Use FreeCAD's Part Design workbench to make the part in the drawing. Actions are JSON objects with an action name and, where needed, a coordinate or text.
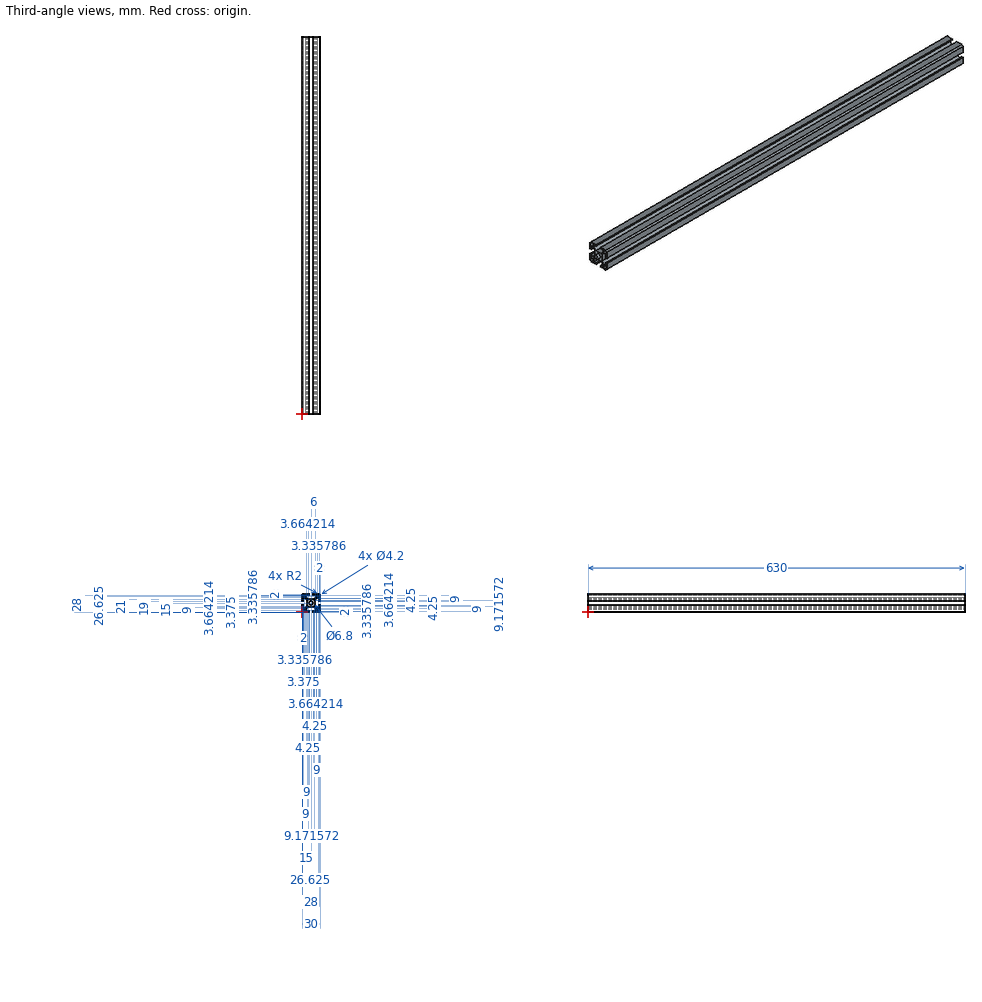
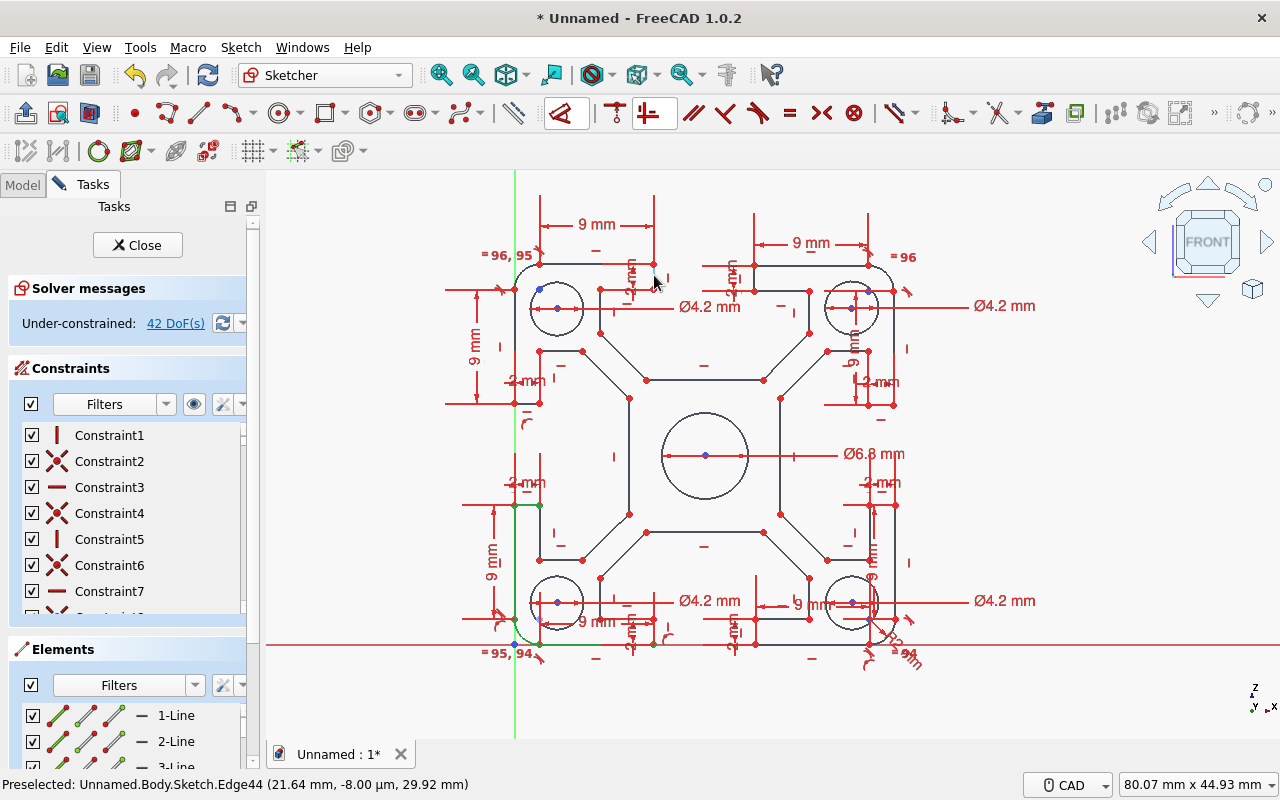
{"action": "left_click", "coordinate": [763, 532]}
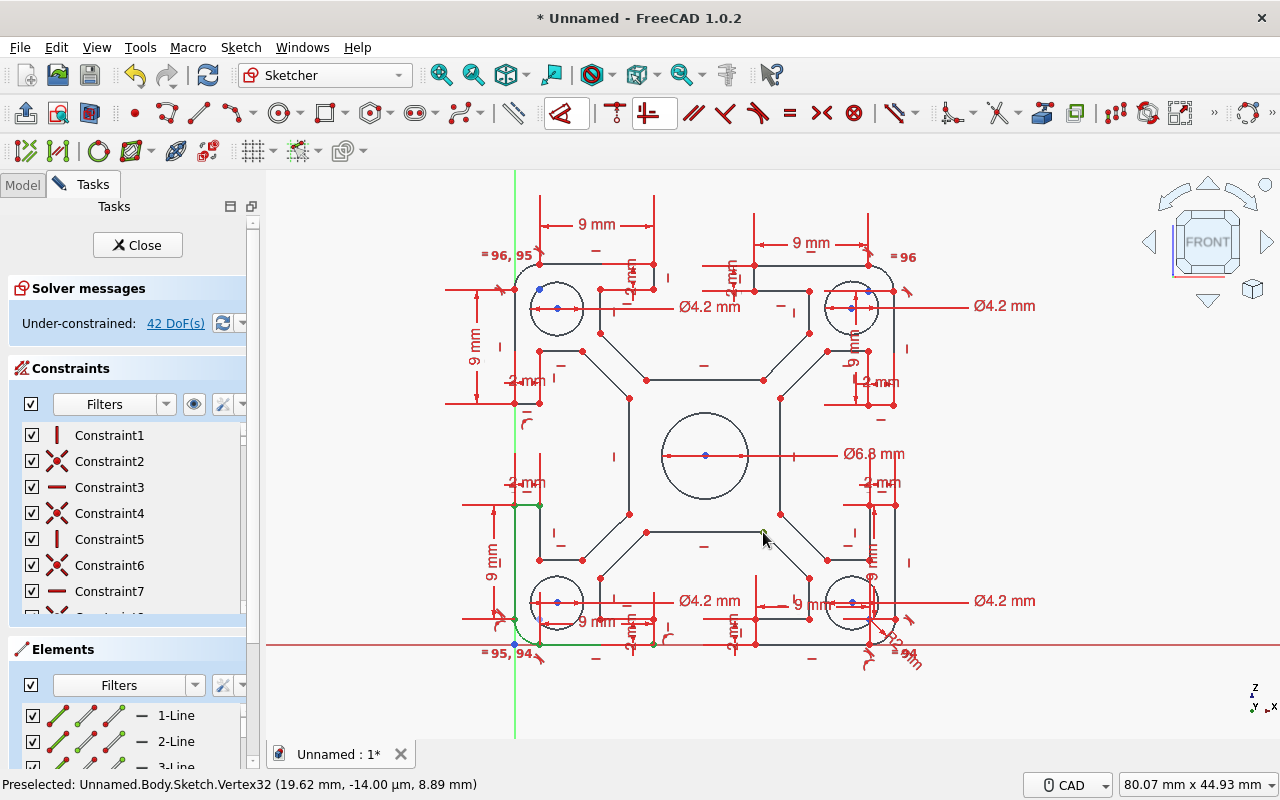
{"action": "key", "text": "i"}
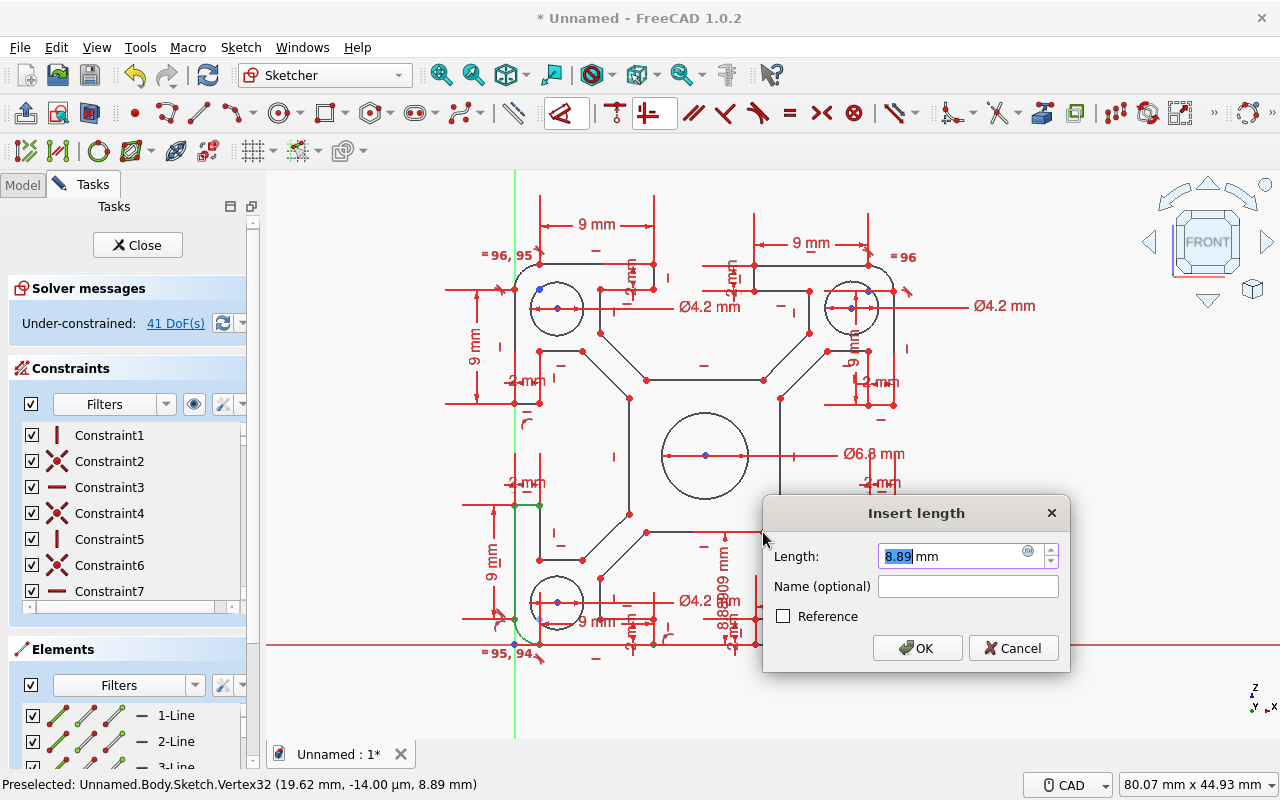
{"action": "type", "text": "9"}
{"action": "key", "text": "Return"}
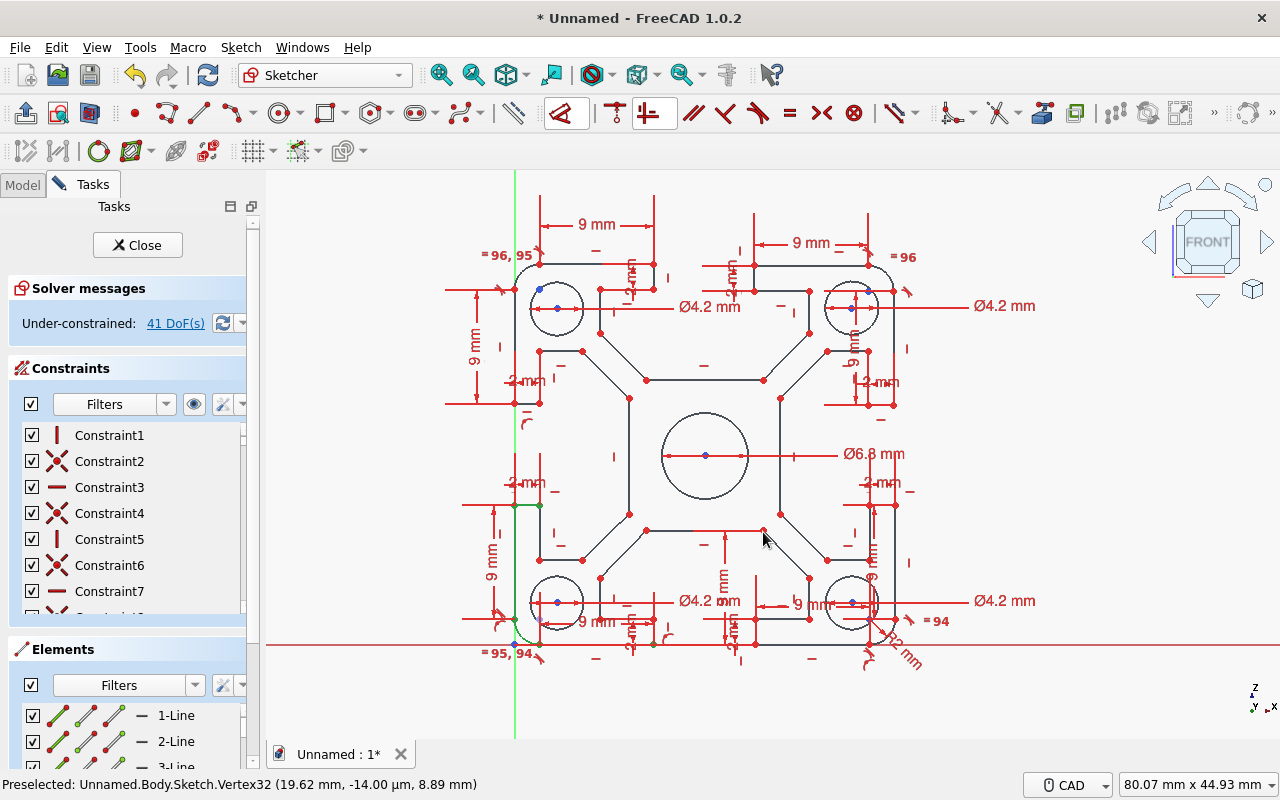
{"action": "left_click", "coordinate": [629, 514]}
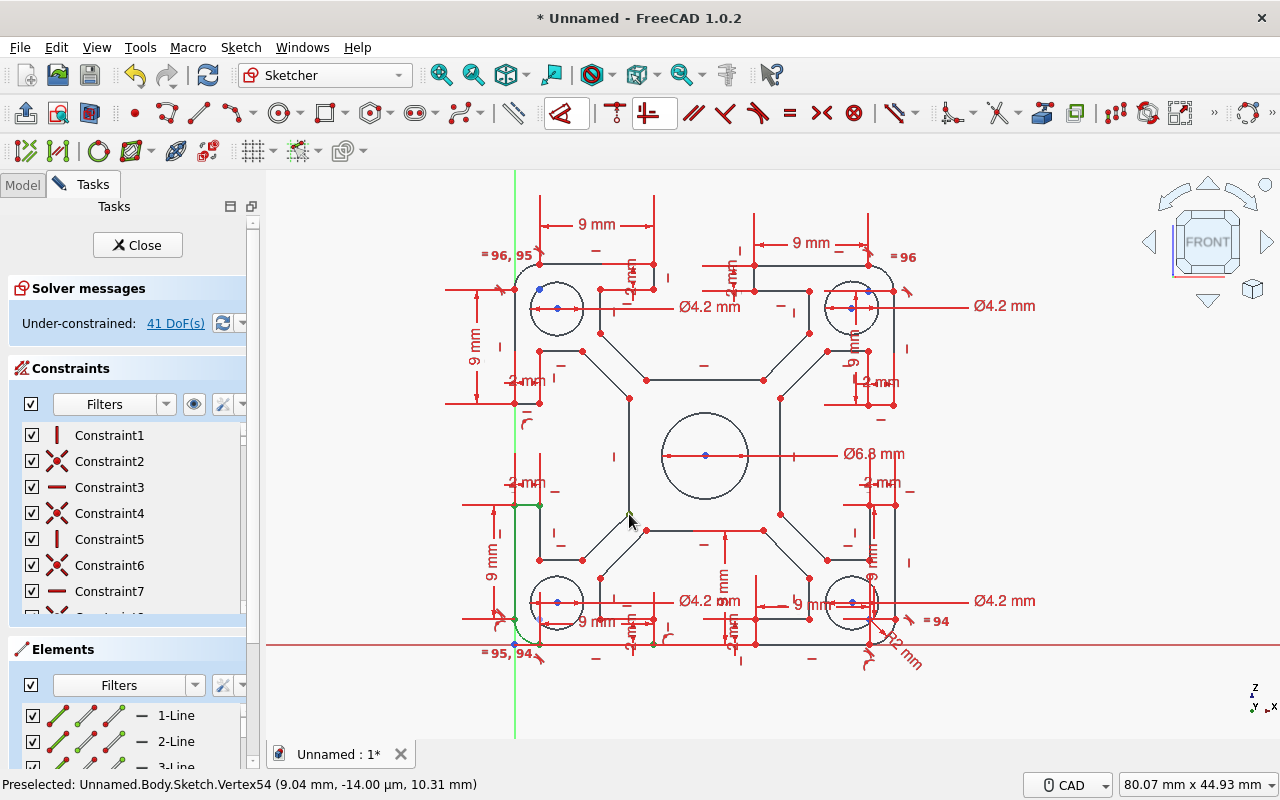
{"action": "left_click", "coordinate": [584, 114]}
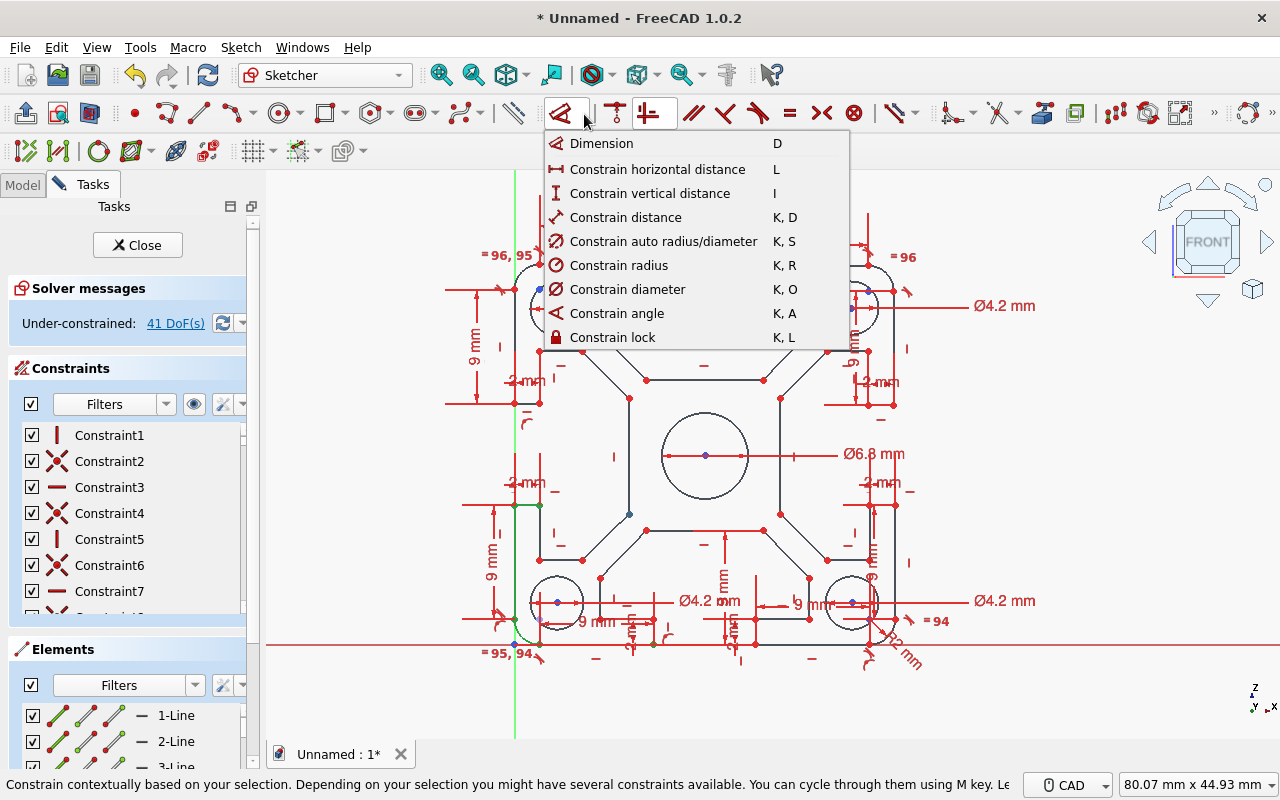
{"action": "left_click", "coordinate": [697, 169]}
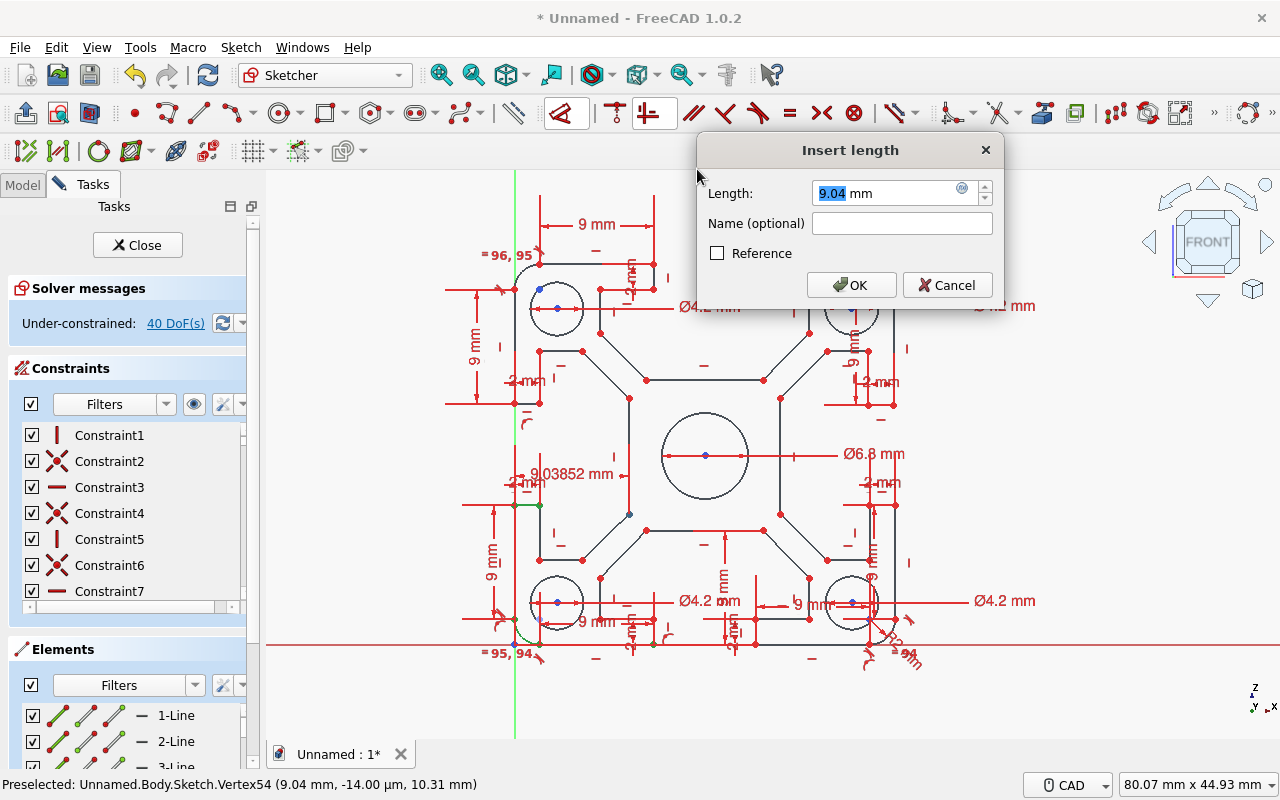
{"action": "type", "text": "9"}
{"action": "key", "text": "Return"}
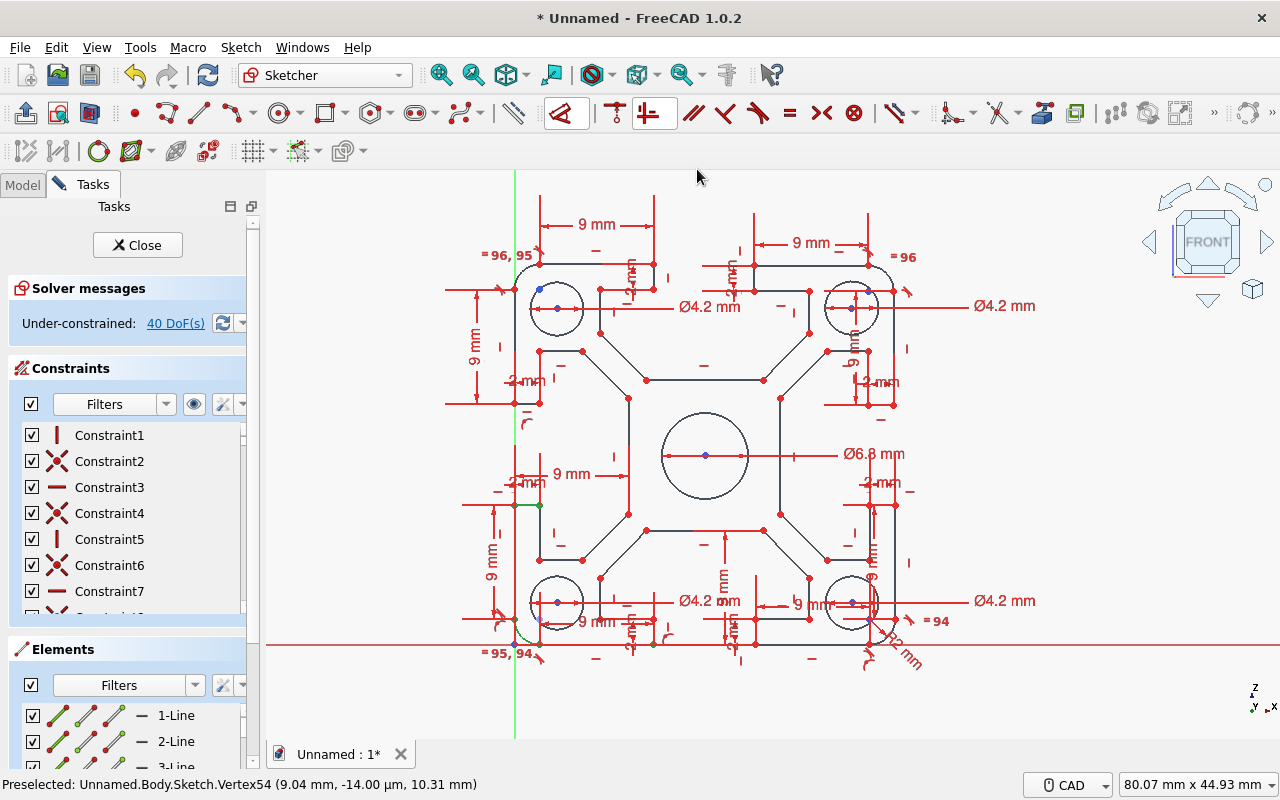
{"action": "left_click", "coordinate": [705, 456]}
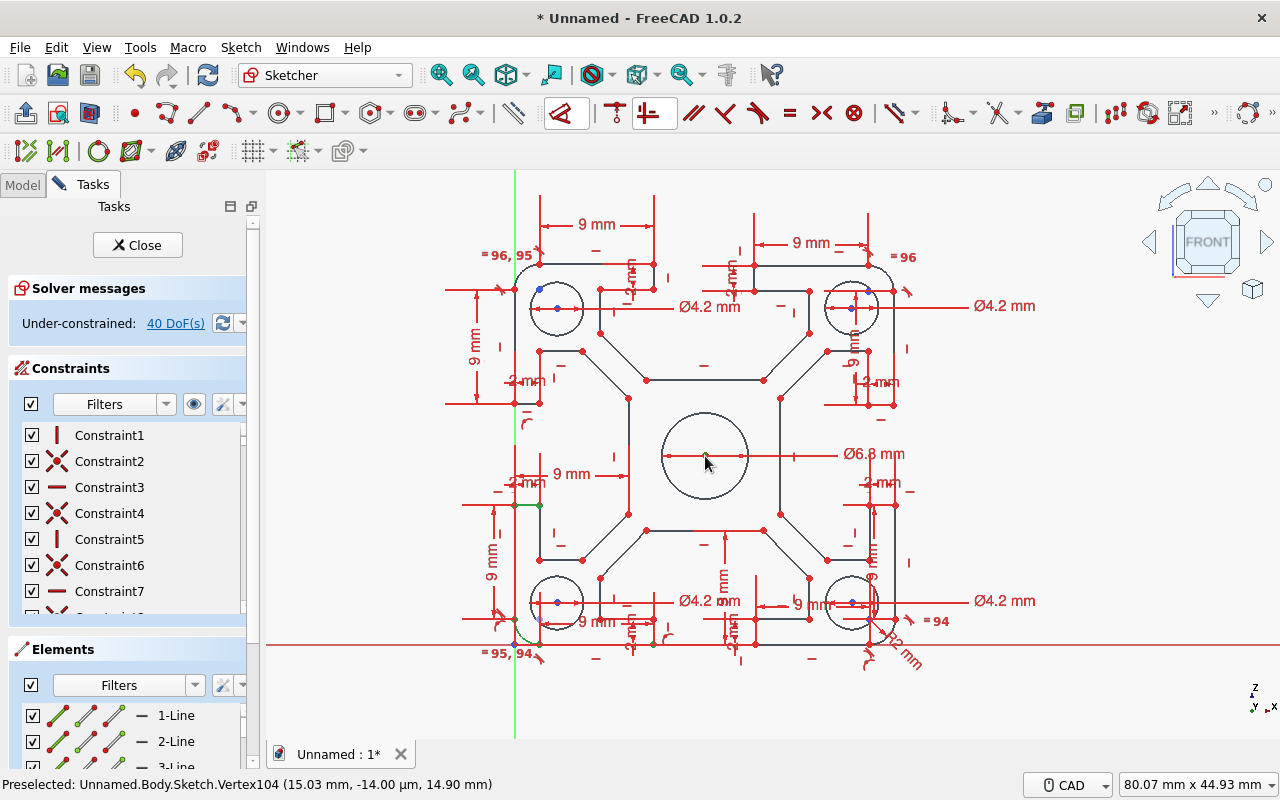
{"action": "key", "text": "l"}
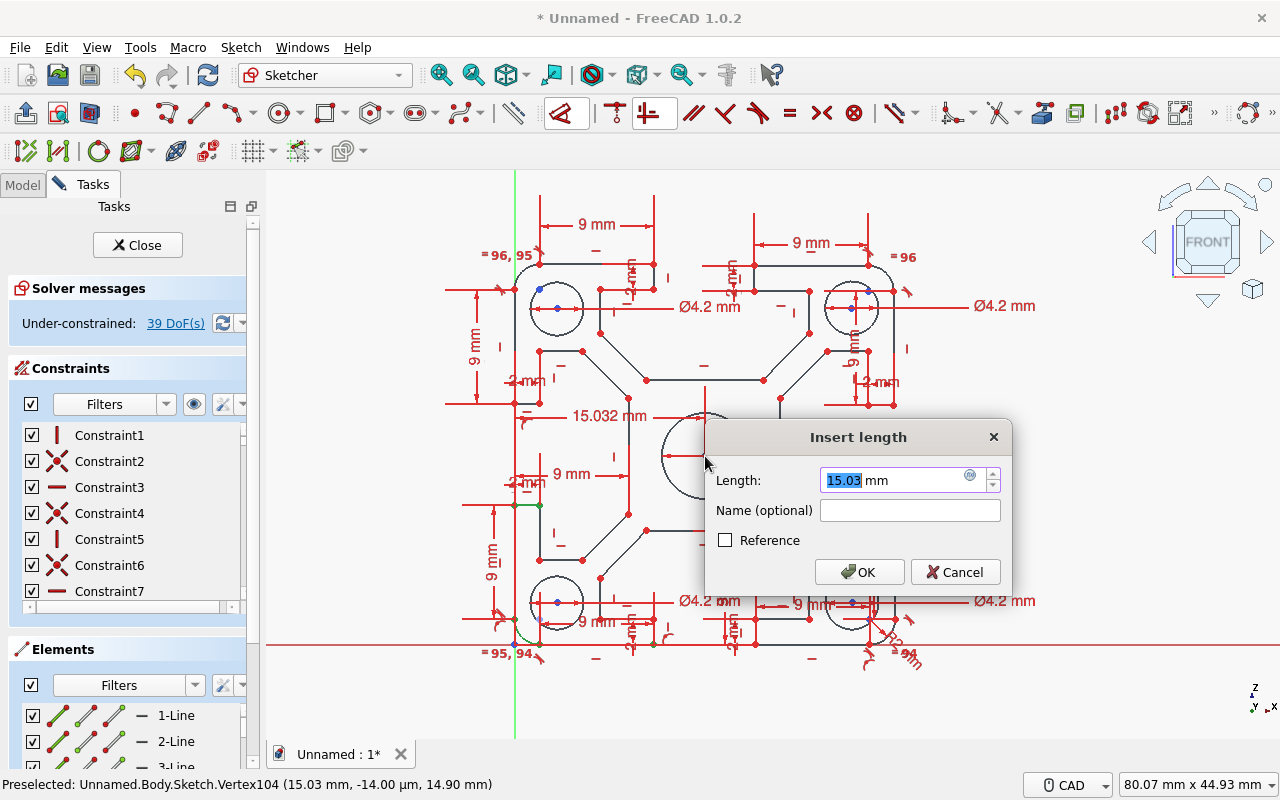
{"action": "type", "text": "15"}
{"action": "key", "text": "Return"}